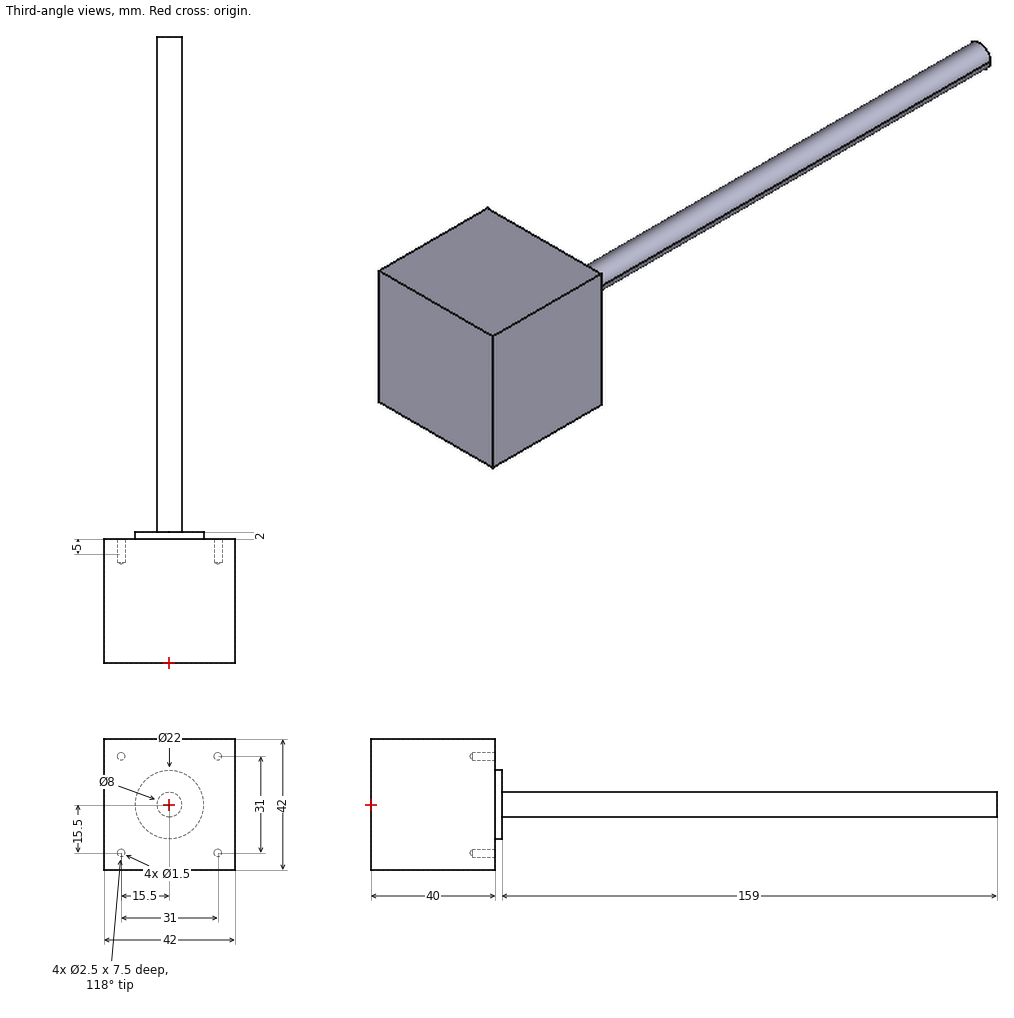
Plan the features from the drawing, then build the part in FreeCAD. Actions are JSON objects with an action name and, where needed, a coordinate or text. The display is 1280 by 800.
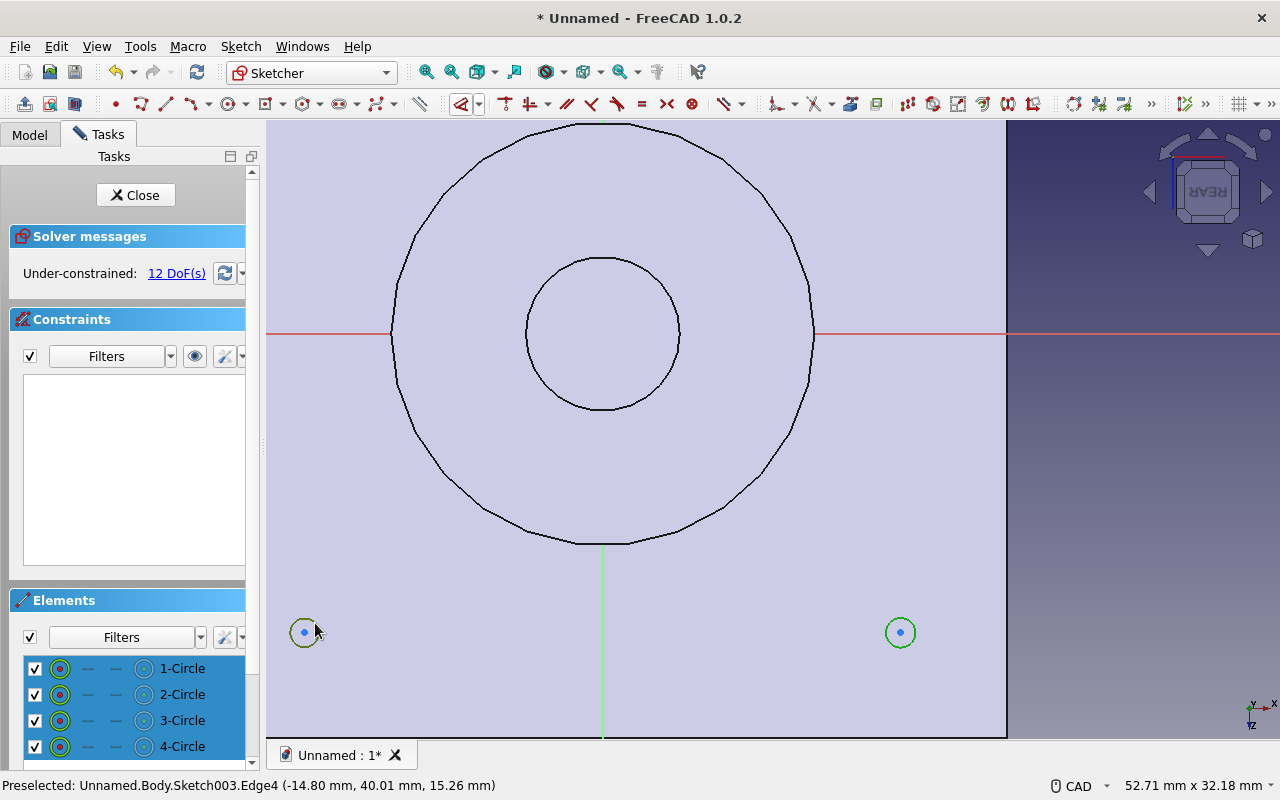
{"action": "key", "text": "e"}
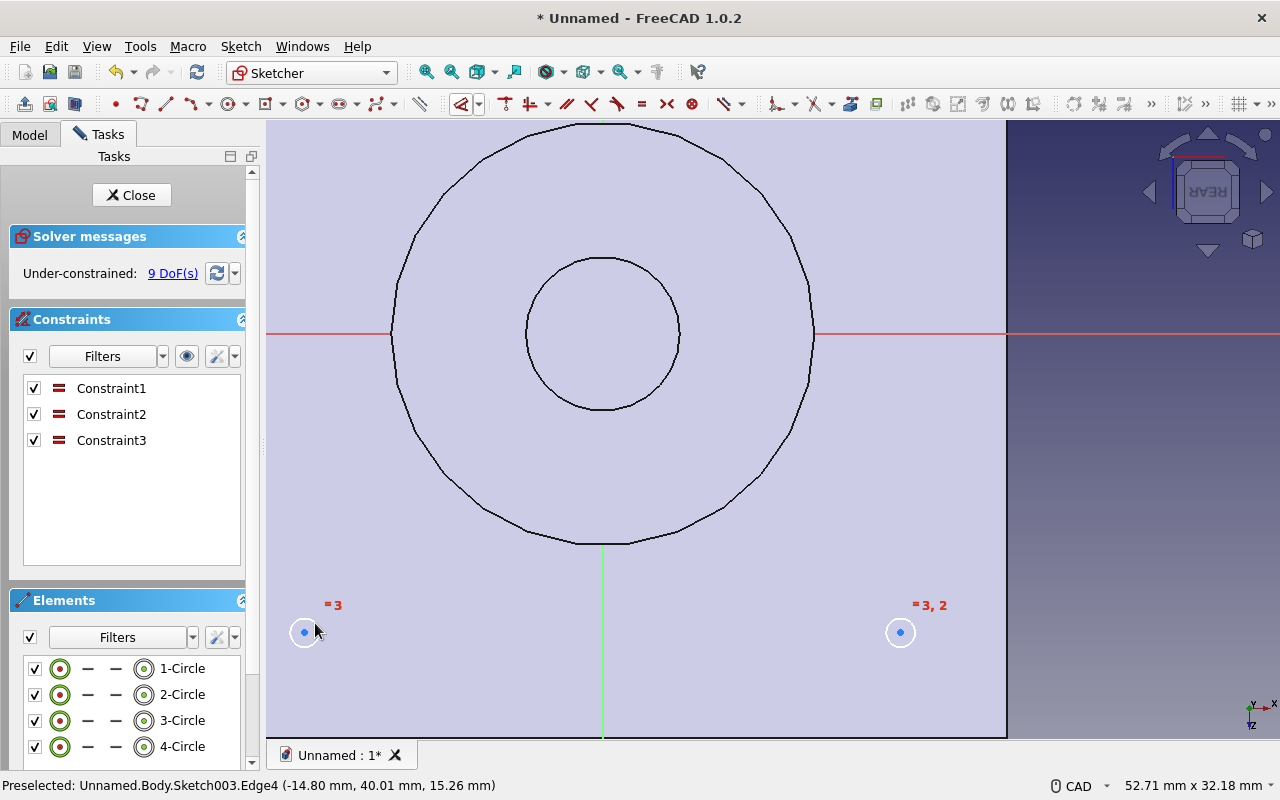
{"action": "scroll", "coordinate": [911, 624], "scroll_direction": "down", "scroll_amount": 2}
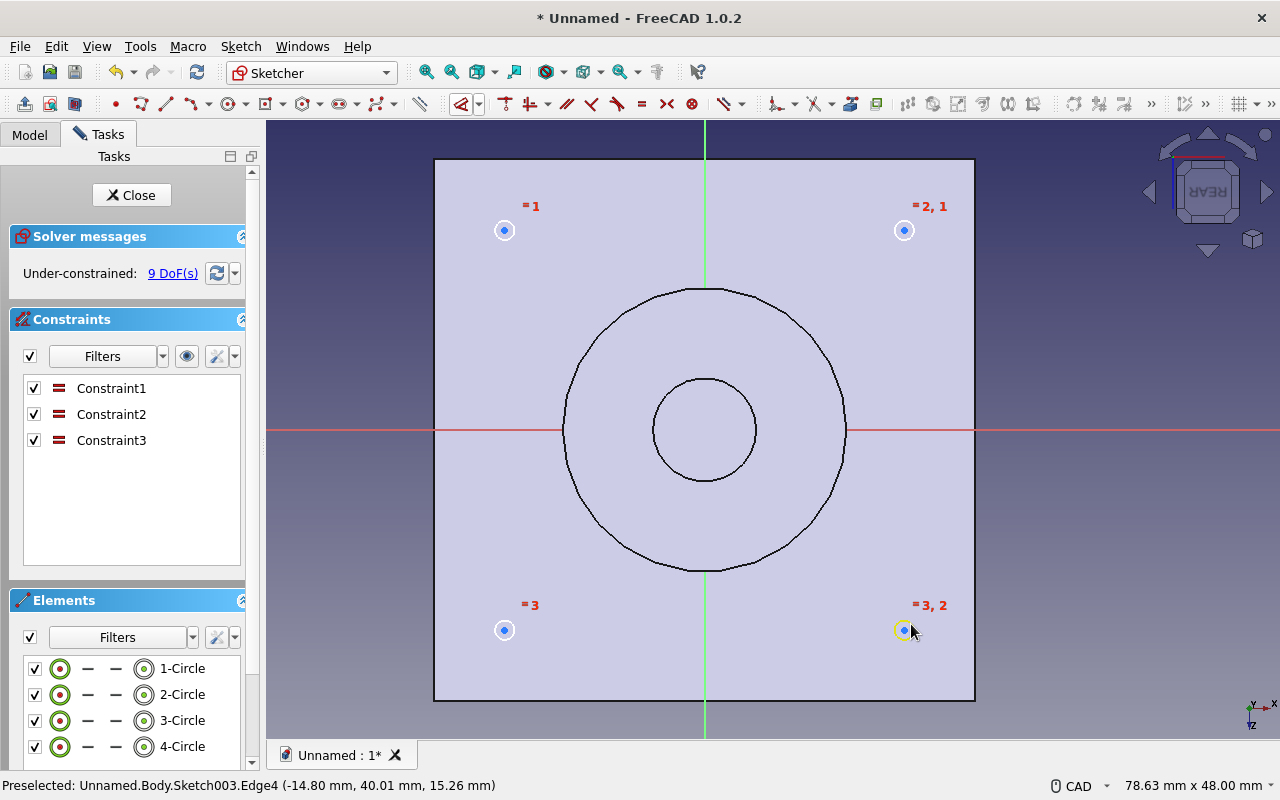
{"action": "left_click", "coordinate": [505, 230]}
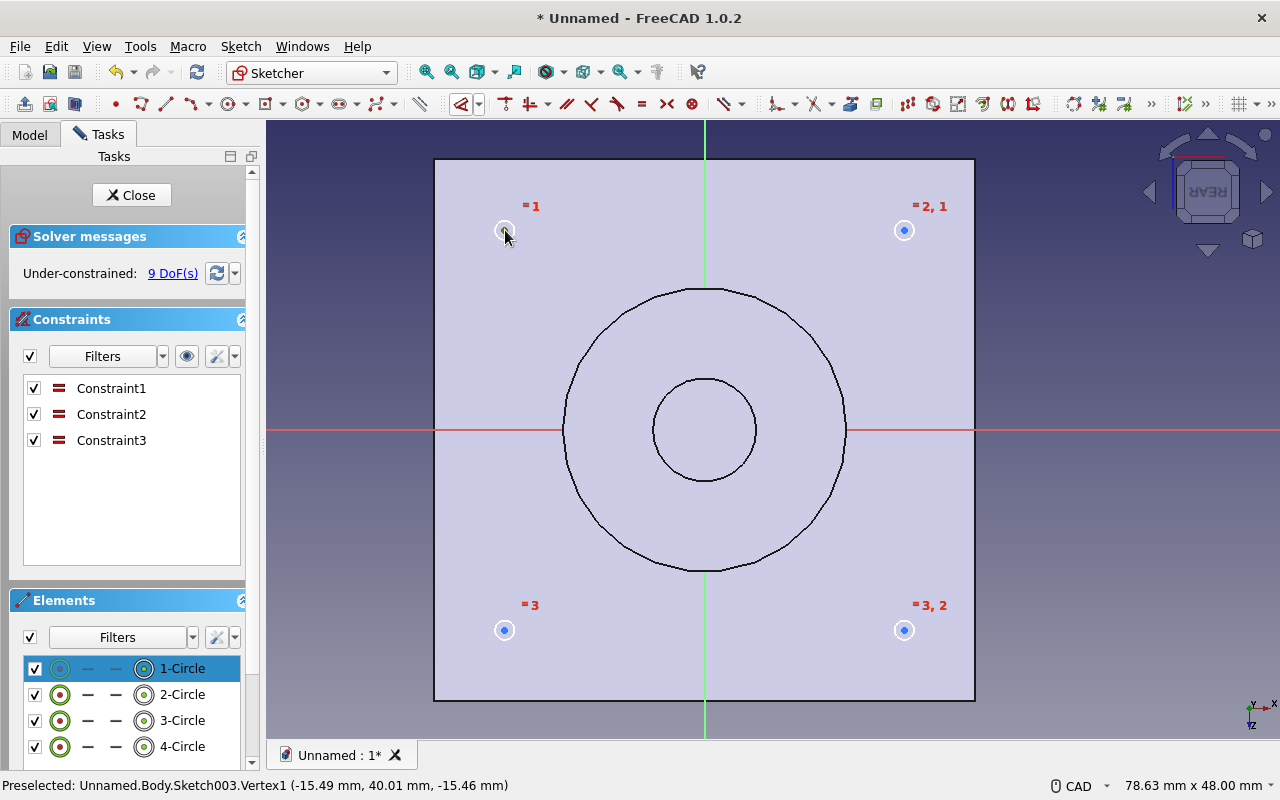
{"action": "left_click", "coordinate": [904, 230]}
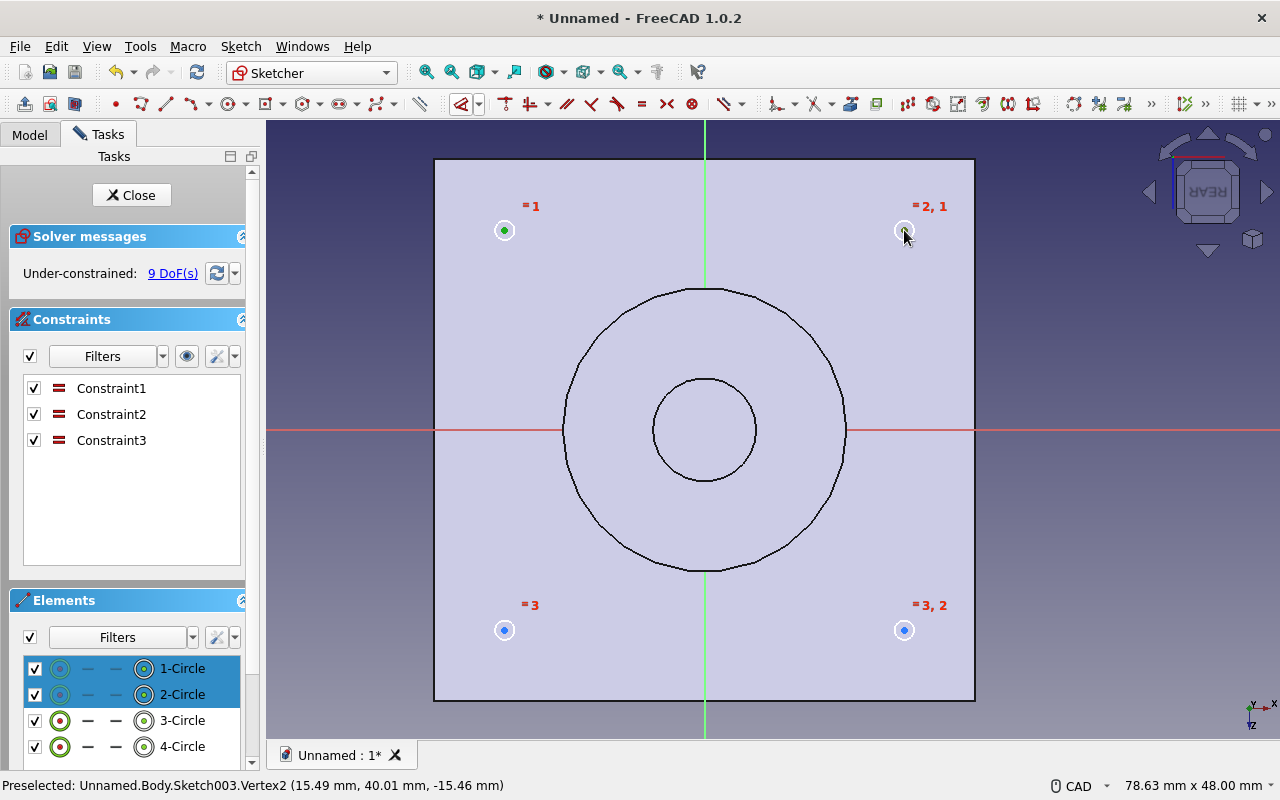
{"action": "key", "text": "h"}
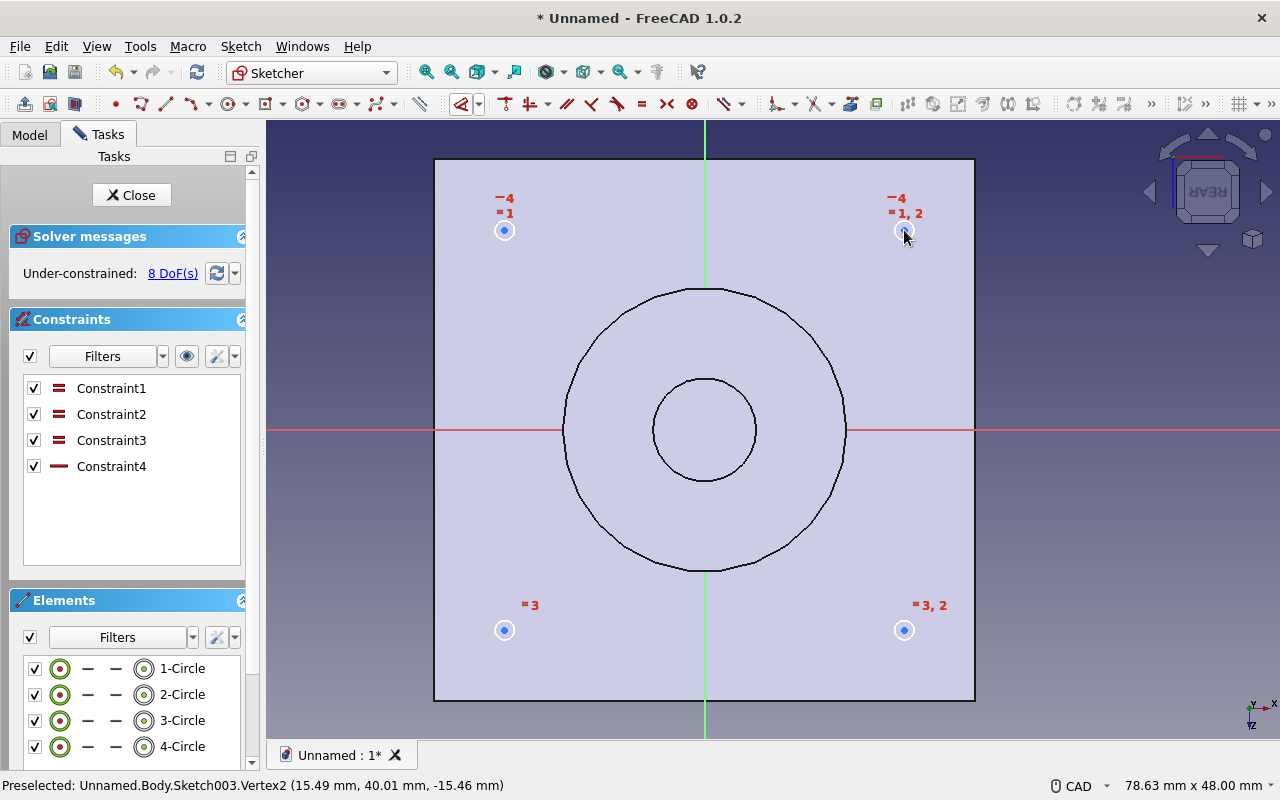
{"action": "left_click", "coordinate": [904, 230]}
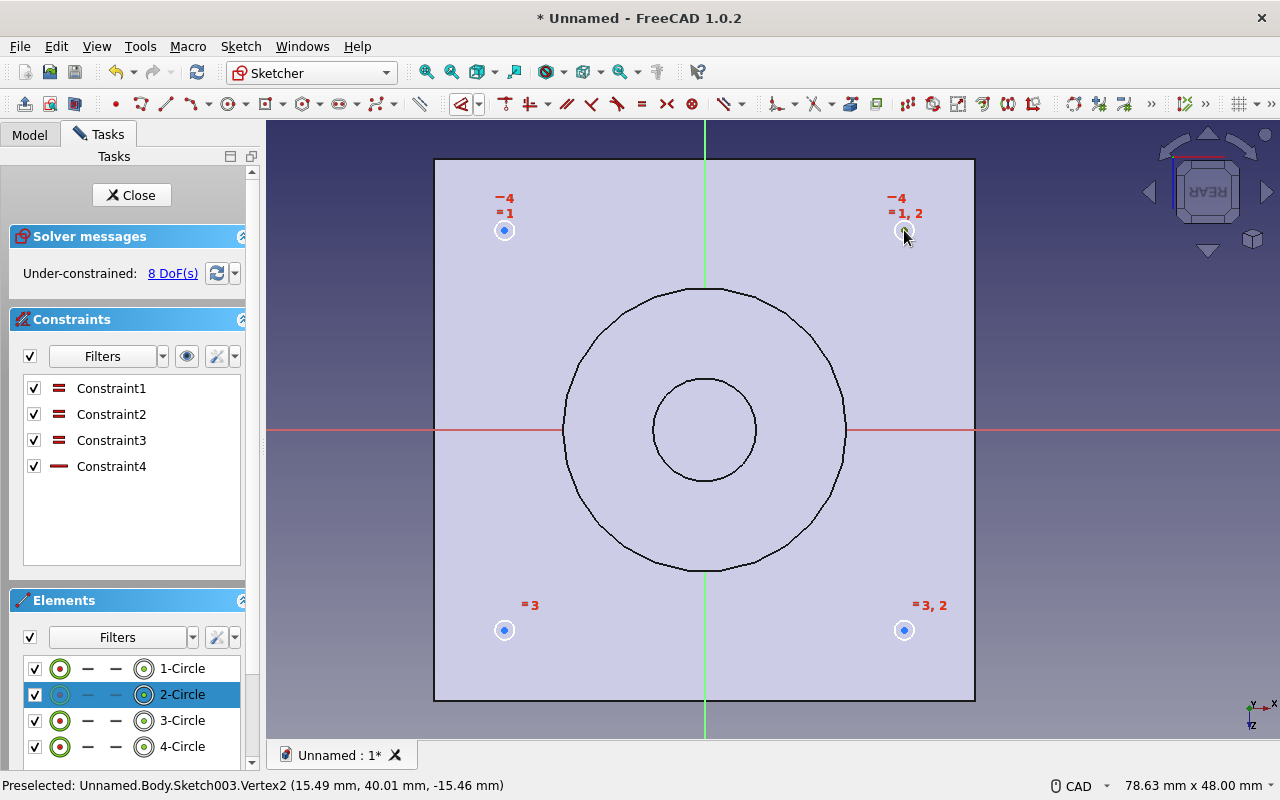
{"action": "left_click", "coordinate": [904, 630]}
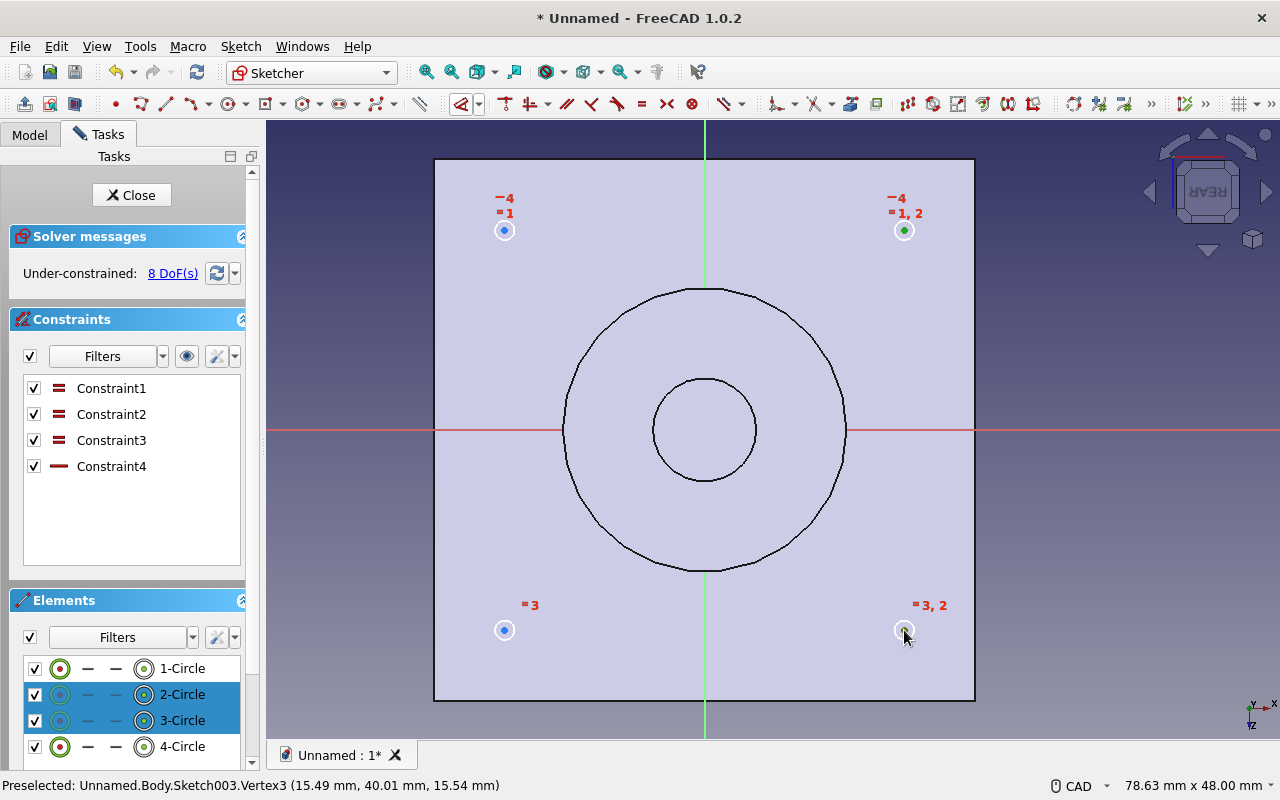
{"action": "key", "text": "v"}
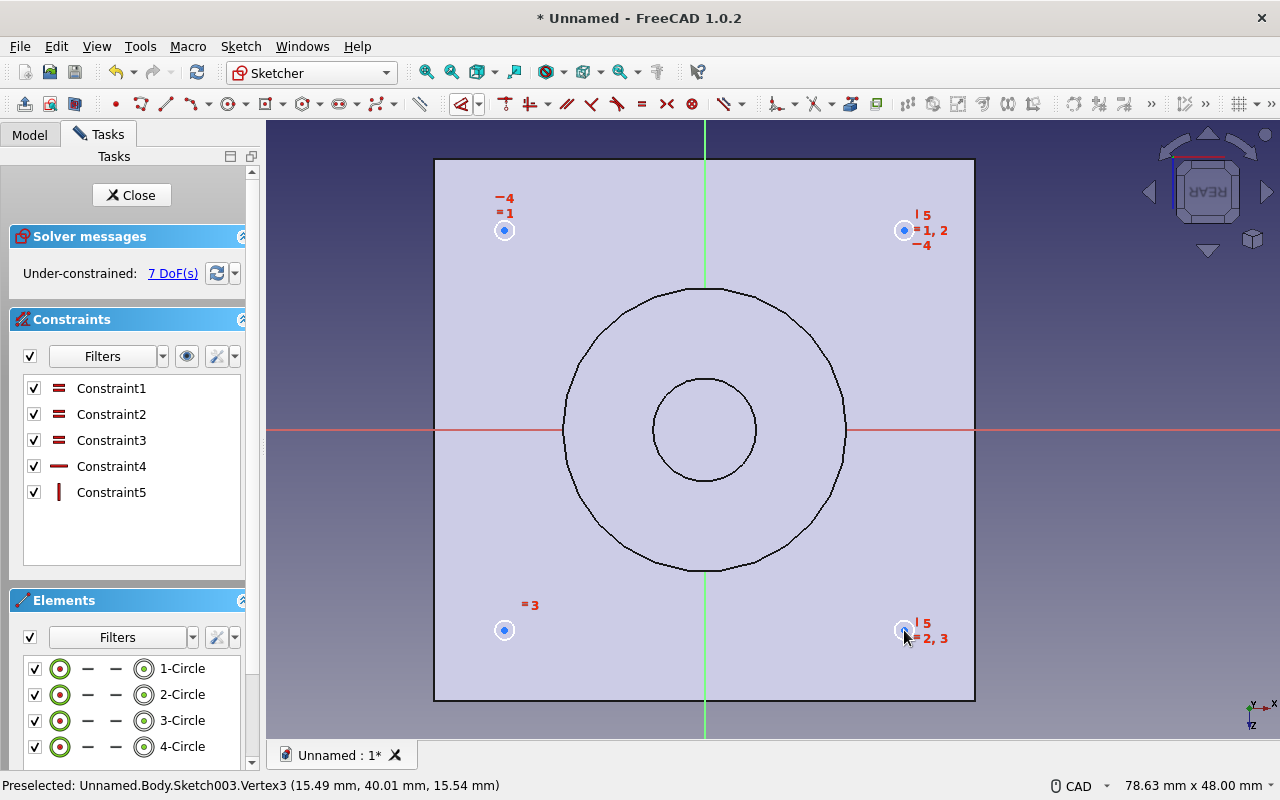
{"action": "left_click", "coordinate": [505, 230]}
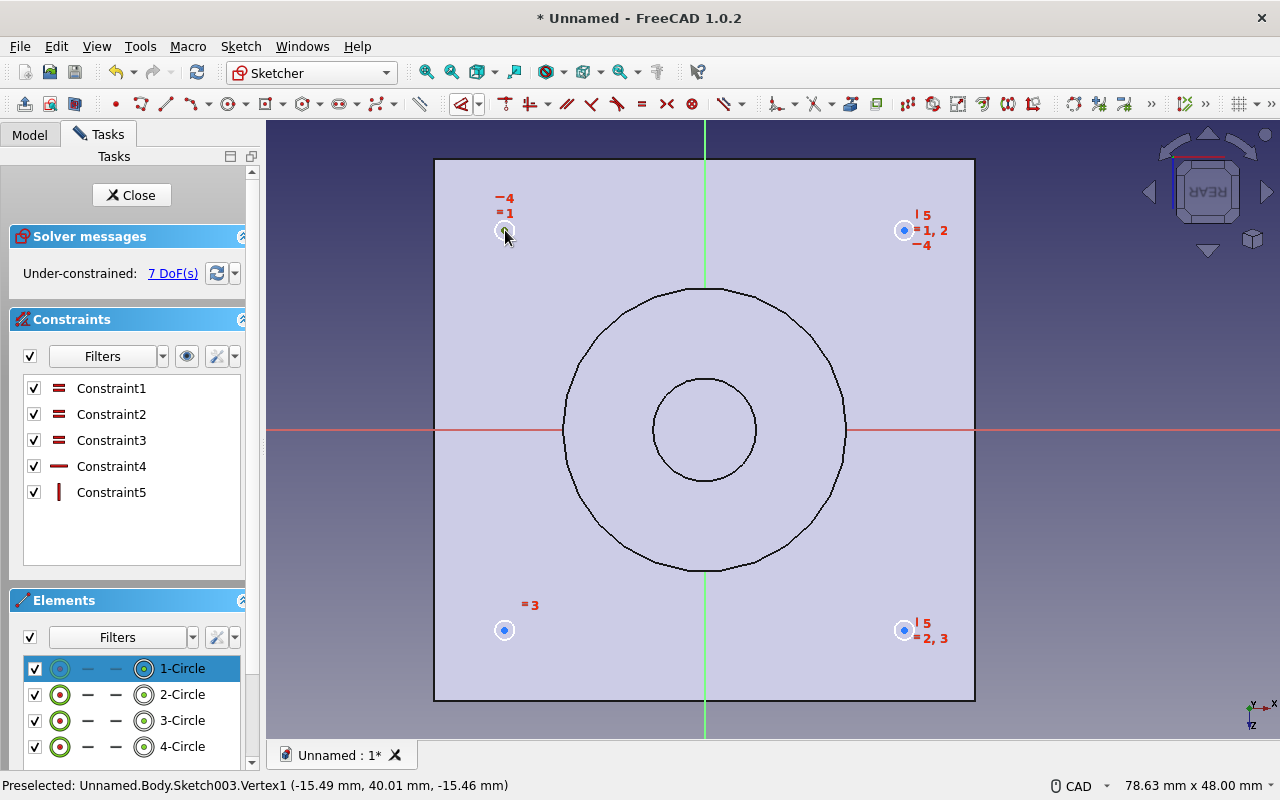
{"action": "left_click", "coordinate": [505, 630]}